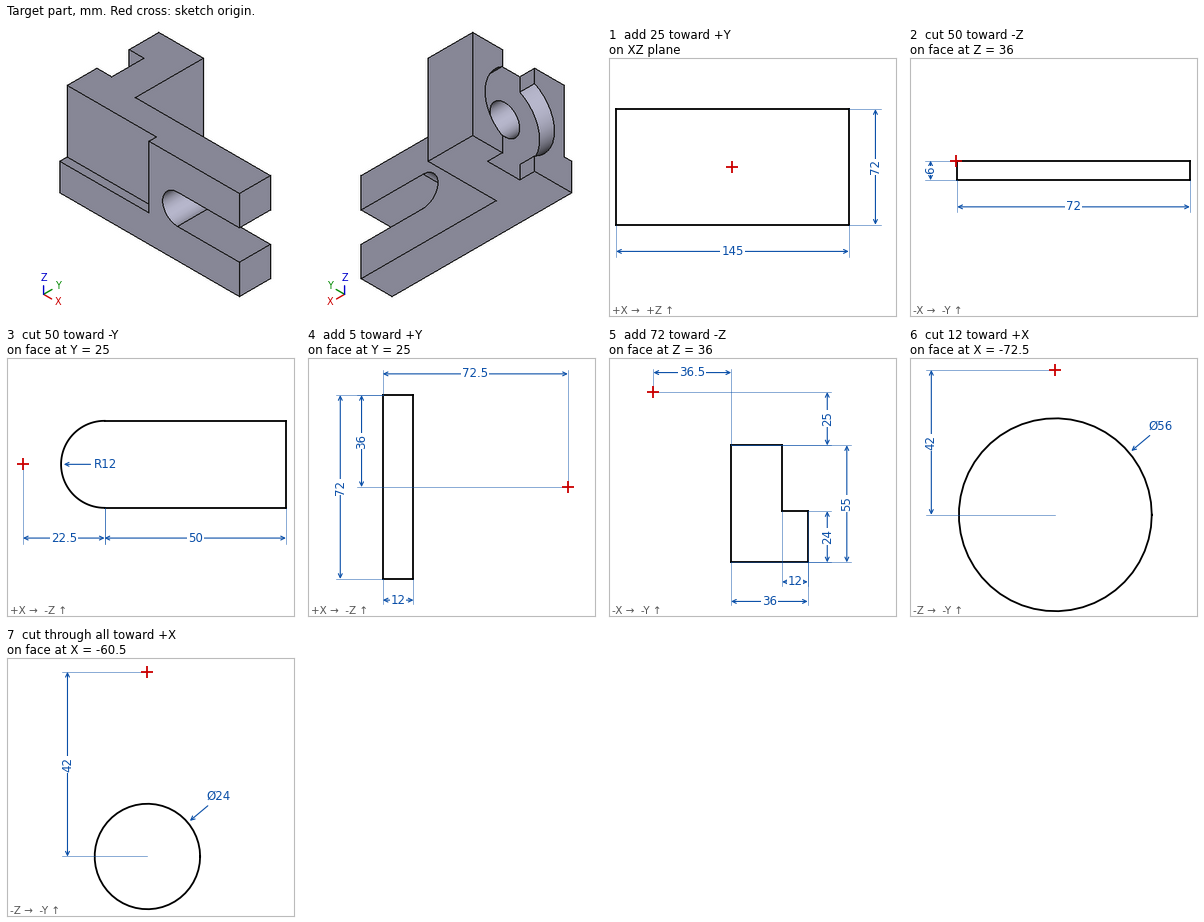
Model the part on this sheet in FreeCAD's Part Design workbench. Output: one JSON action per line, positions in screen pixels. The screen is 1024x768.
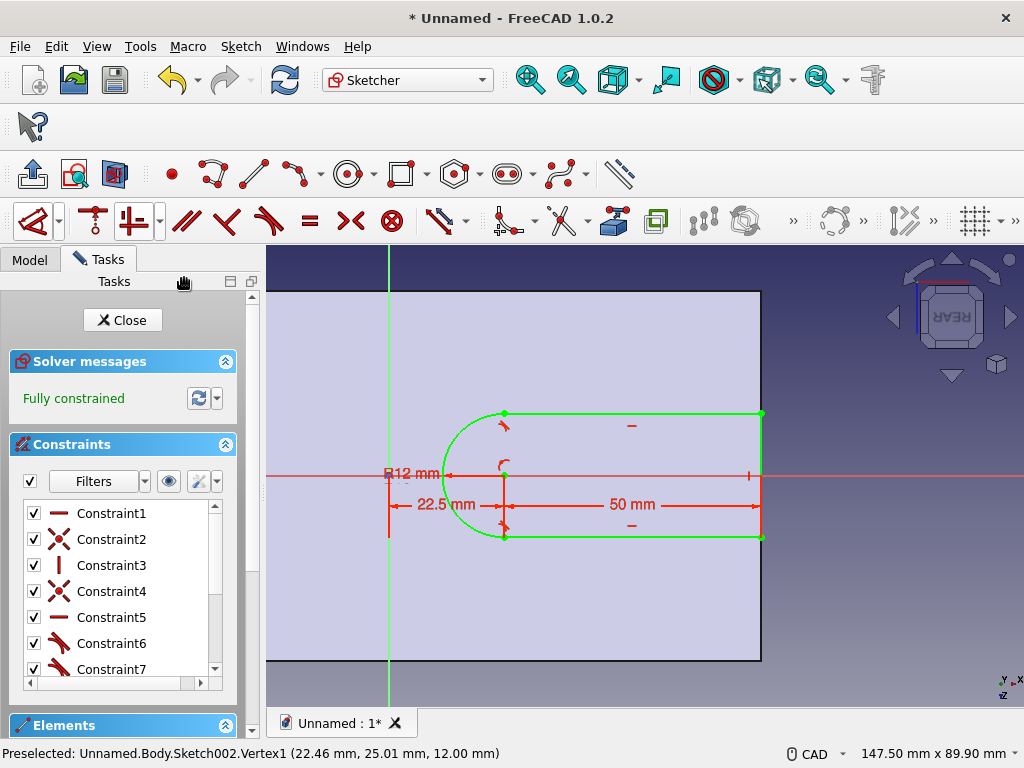
{"action": "left_click", "coordinate": [123, 320]}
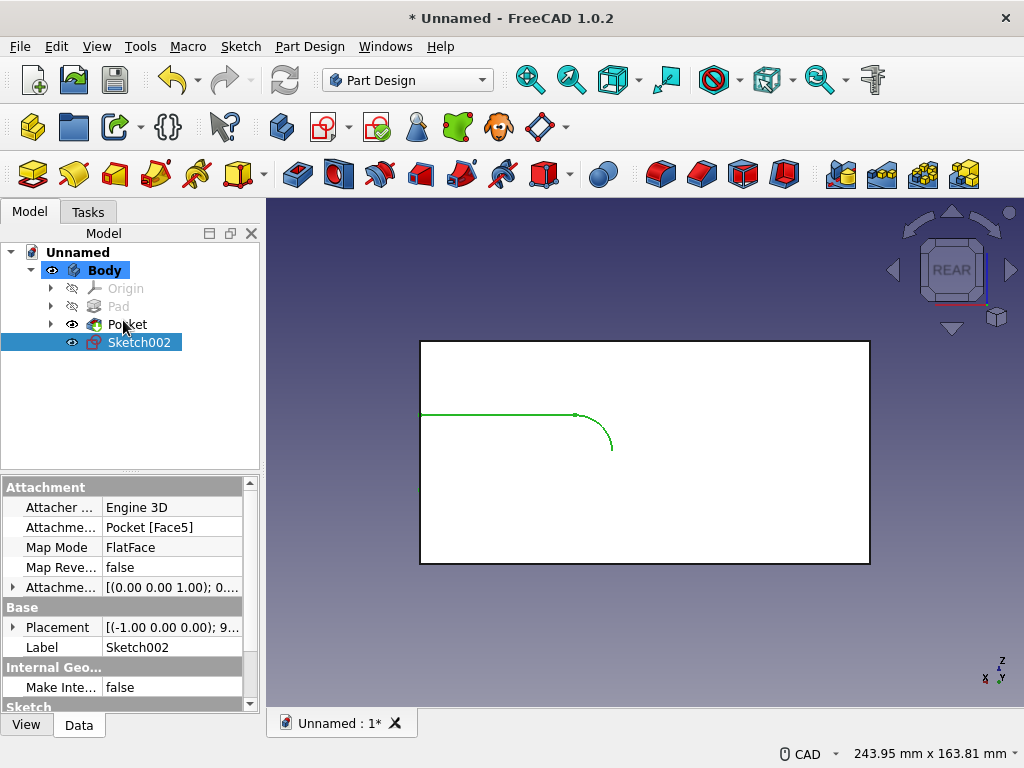
{"action": "left_click", "coordinate": [298, 174]}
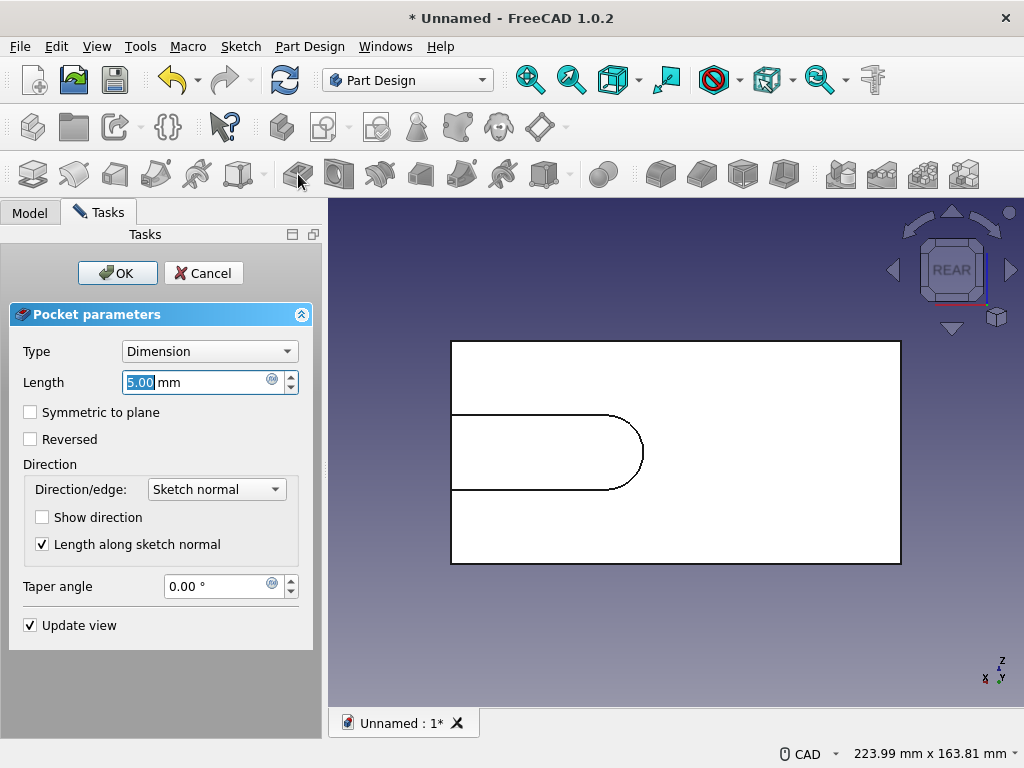
{"action": "type", "text": "50"}
{"action": "key", "text": "Tab"}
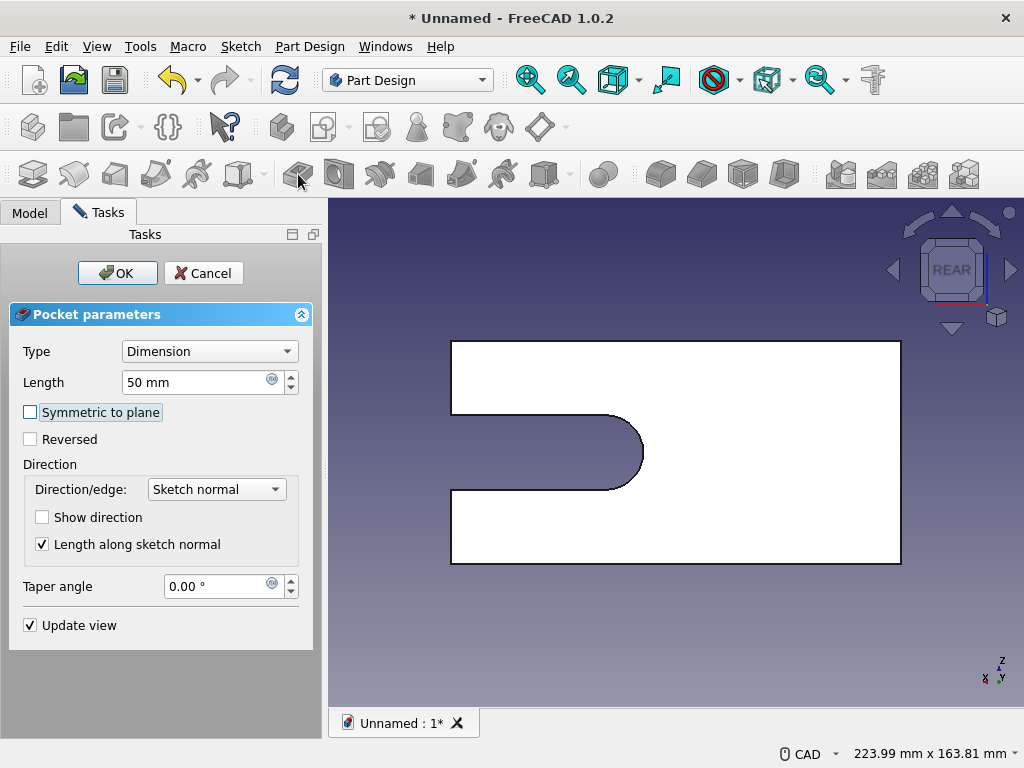
{"action": "left_click", "coordinate": [118, 273]}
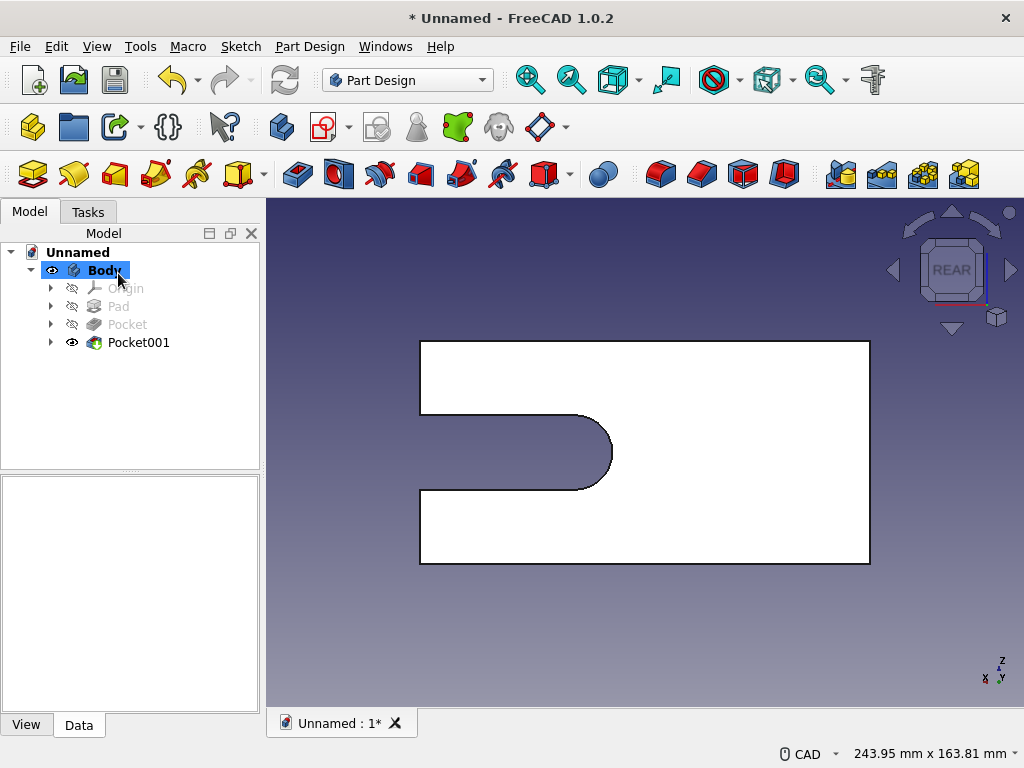
{"action": "left_click", "coordinate": [709, 452]}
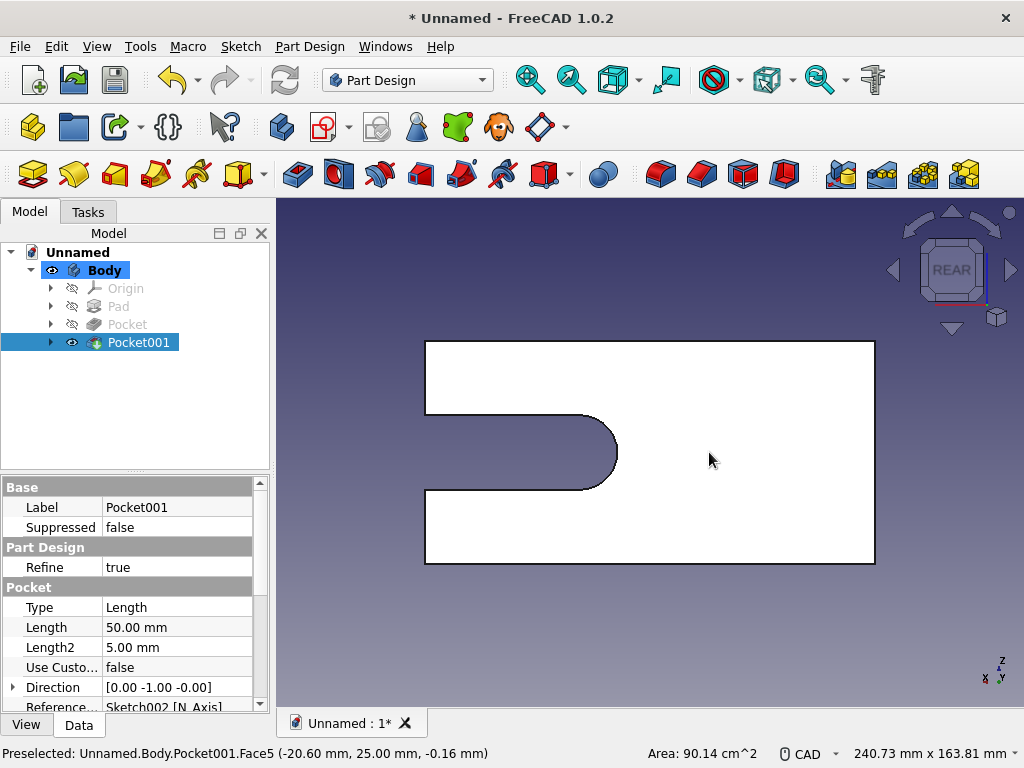
{"action": "left_click", "coordinate": [322, 128]}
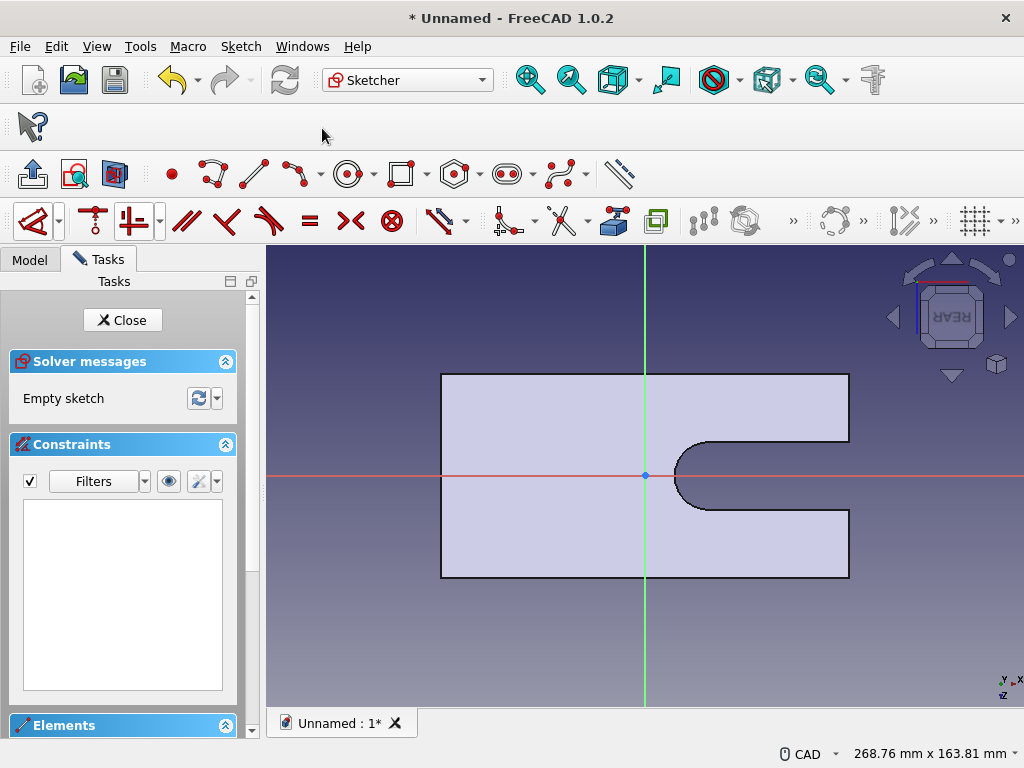
{"action": "scroll", "coordinate": [474, 476], "scroll_direction": "up", "scroll_amount": 2}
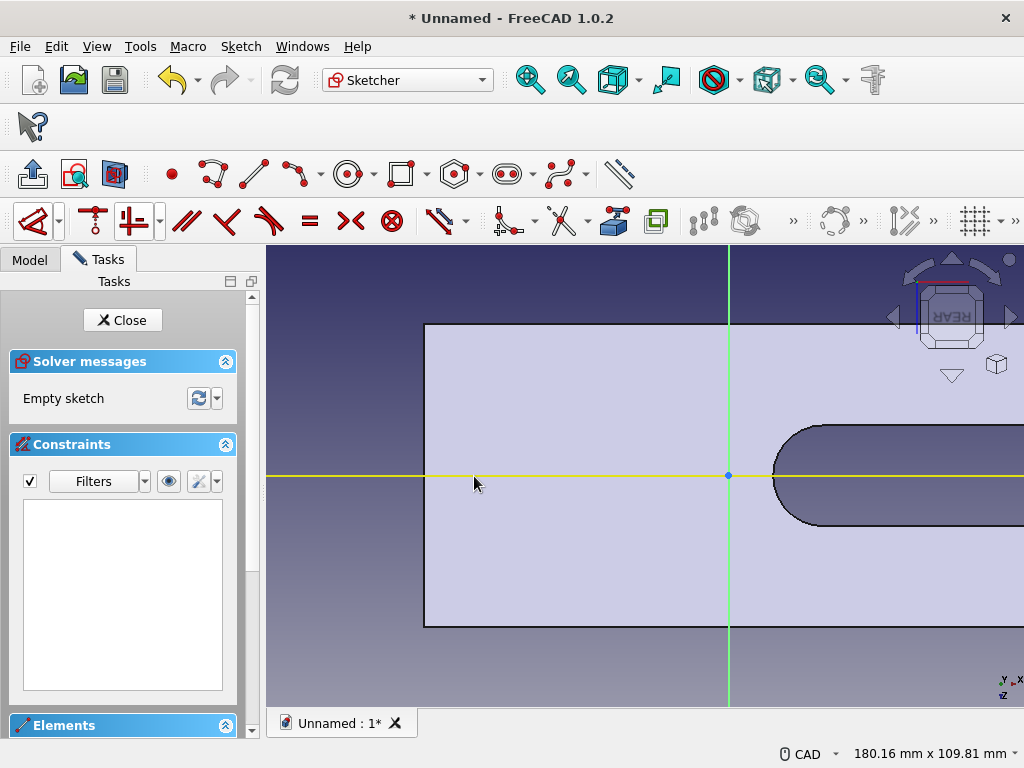
{"action": "left_click", "coordinate": [400, 174]}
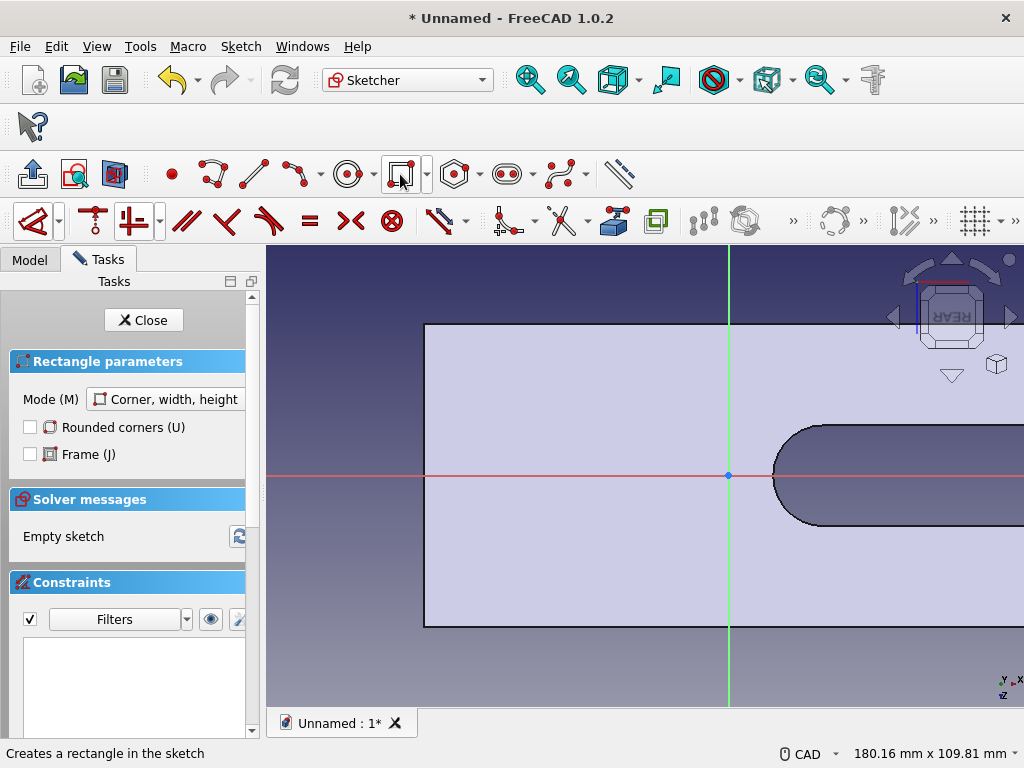
{"action": "left_click", "coordinate": [424, 324]}
{"action": "left_click", "coordinate": [474, 627]}
{"action": "key", "text": "Escape"}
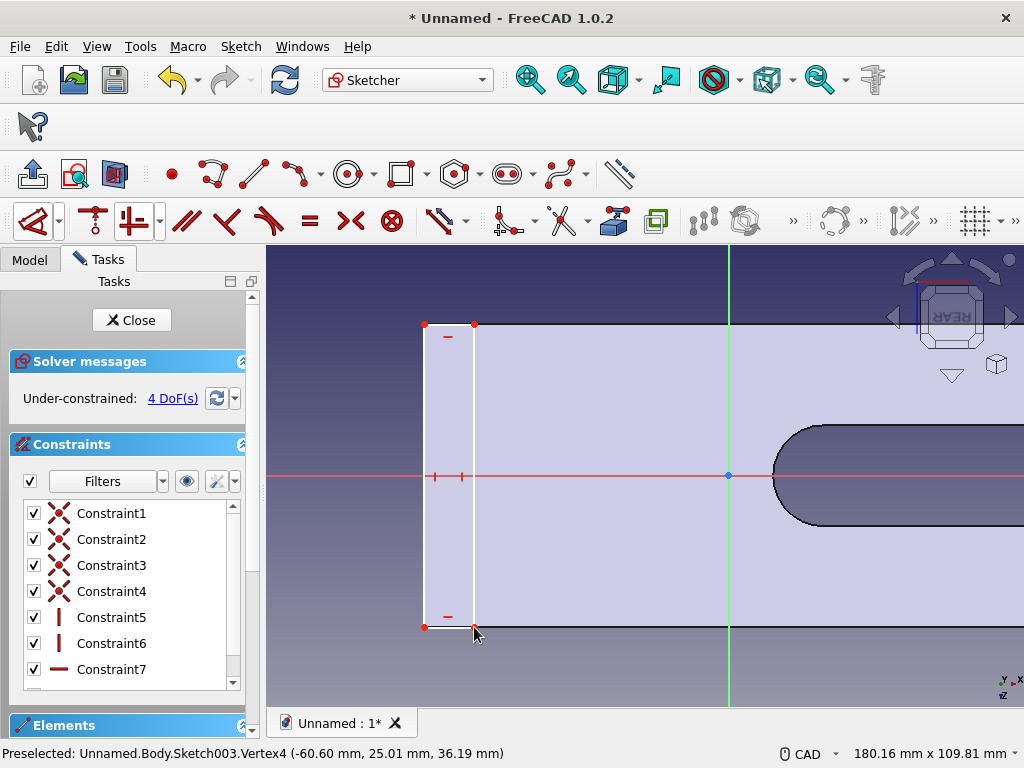
{"action": "left_click", "coordinate": [424, 416]}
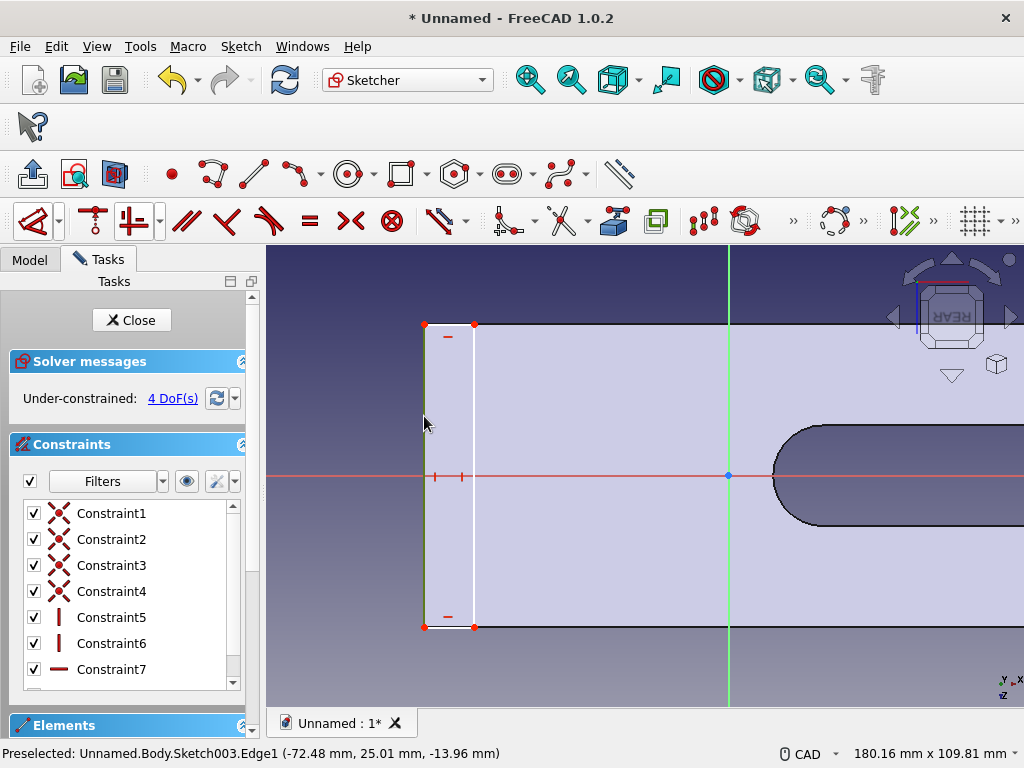
{"action": "key", "text": "i"}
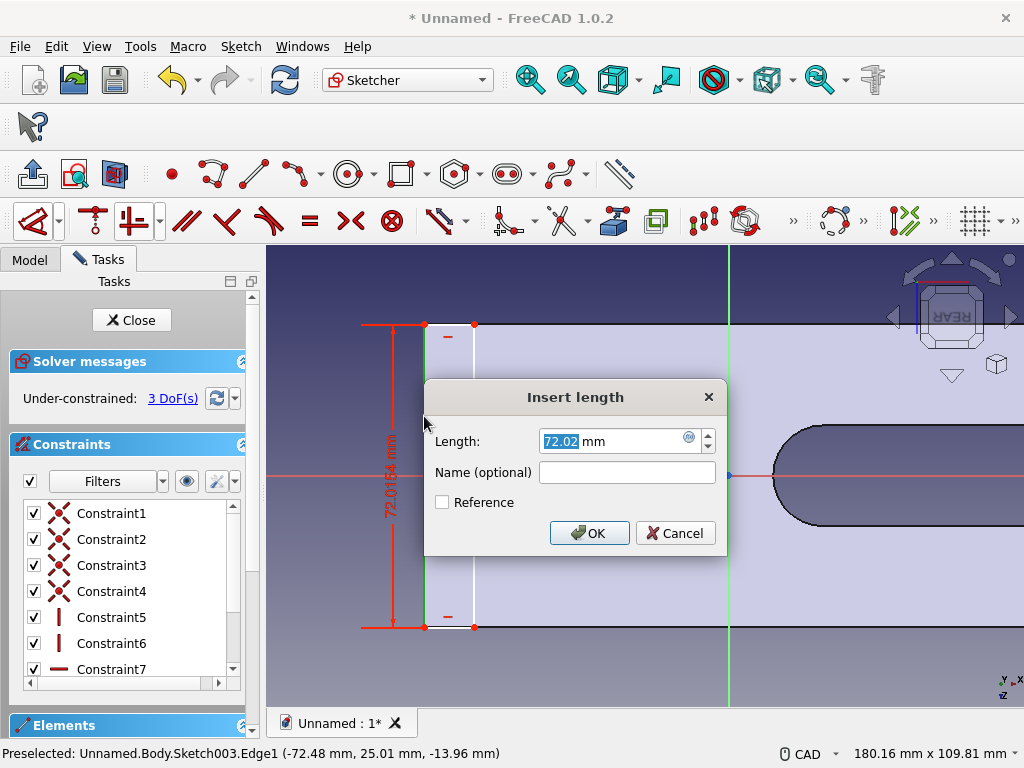
{"action": "type", "text": "72"}
{"action": "key", "text": "Return"}